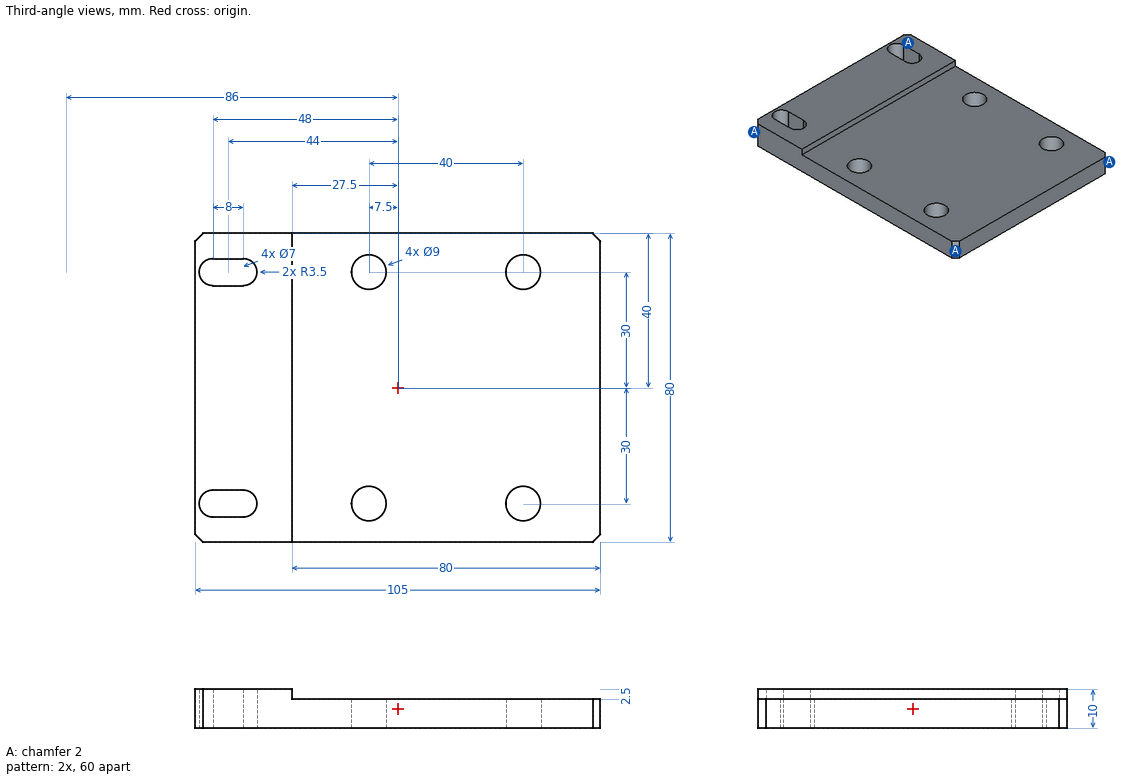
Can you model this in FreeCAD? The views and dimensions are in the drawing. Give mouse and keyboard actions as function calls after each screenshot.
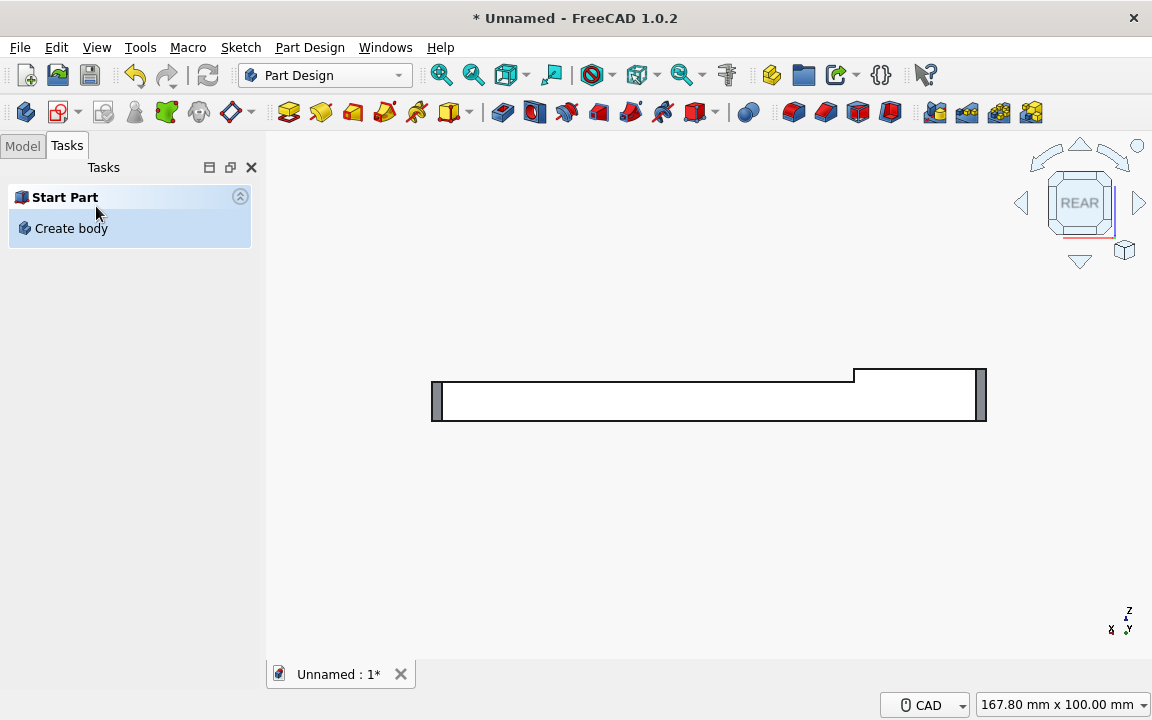
key(0)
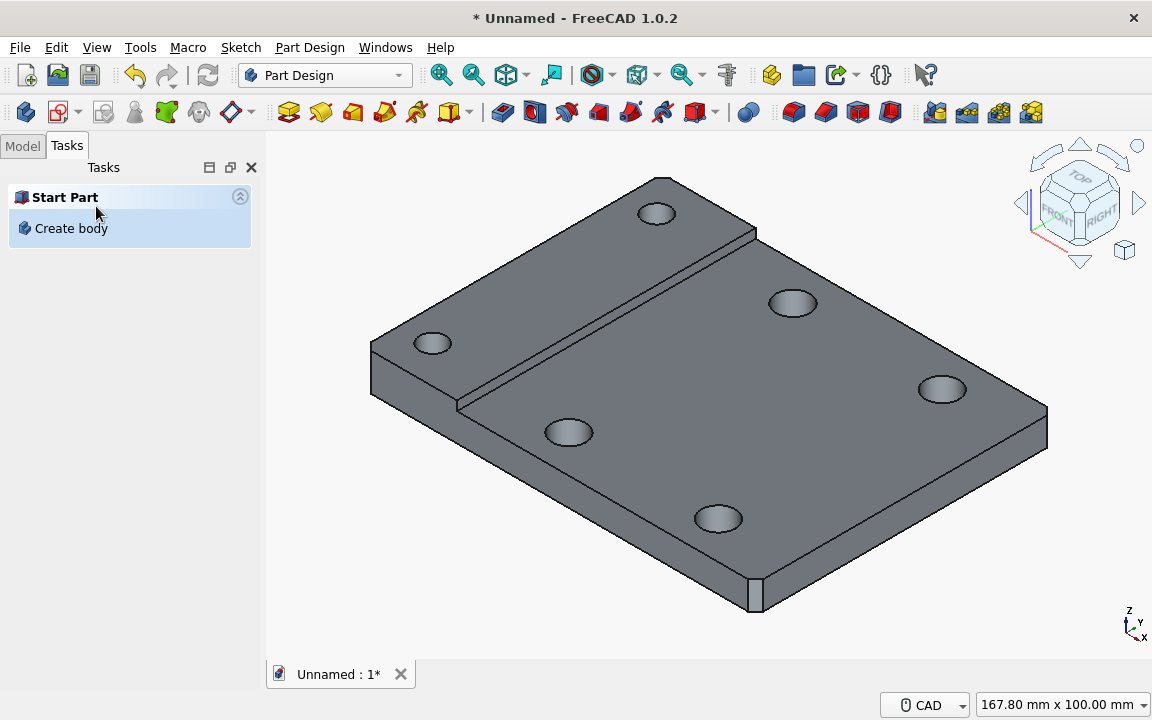
click(602, 262)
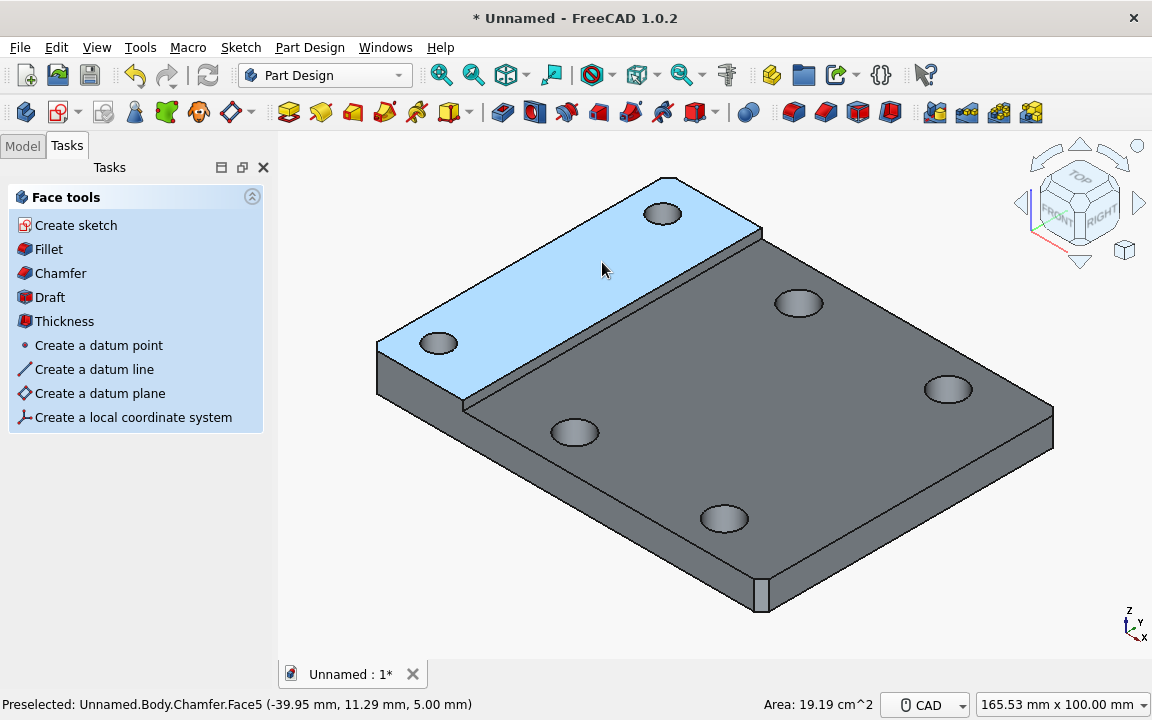
click(58, 112)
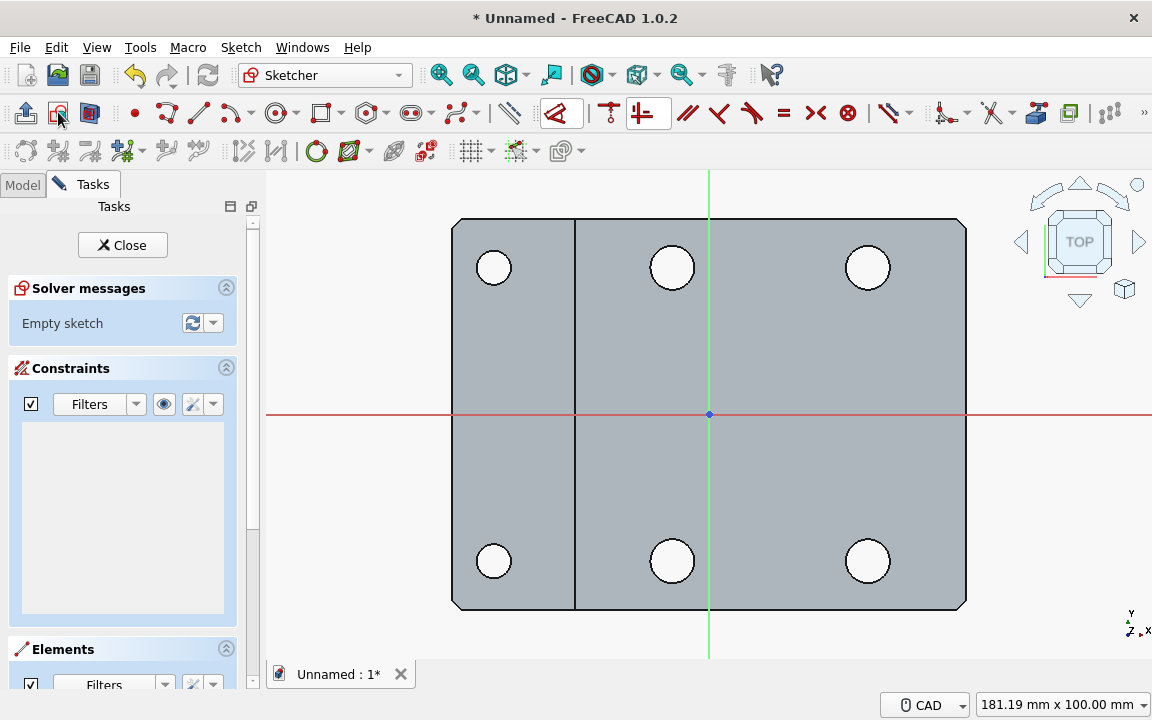
scroll(465, 239, up, 9)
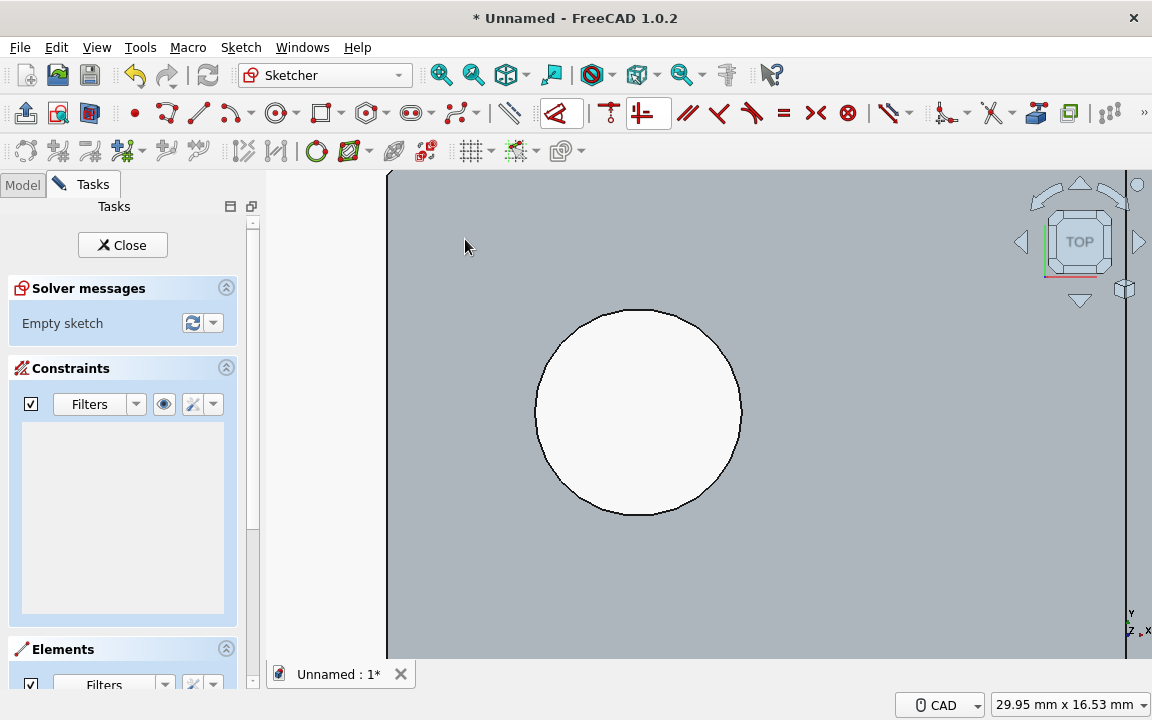
click(412, 114)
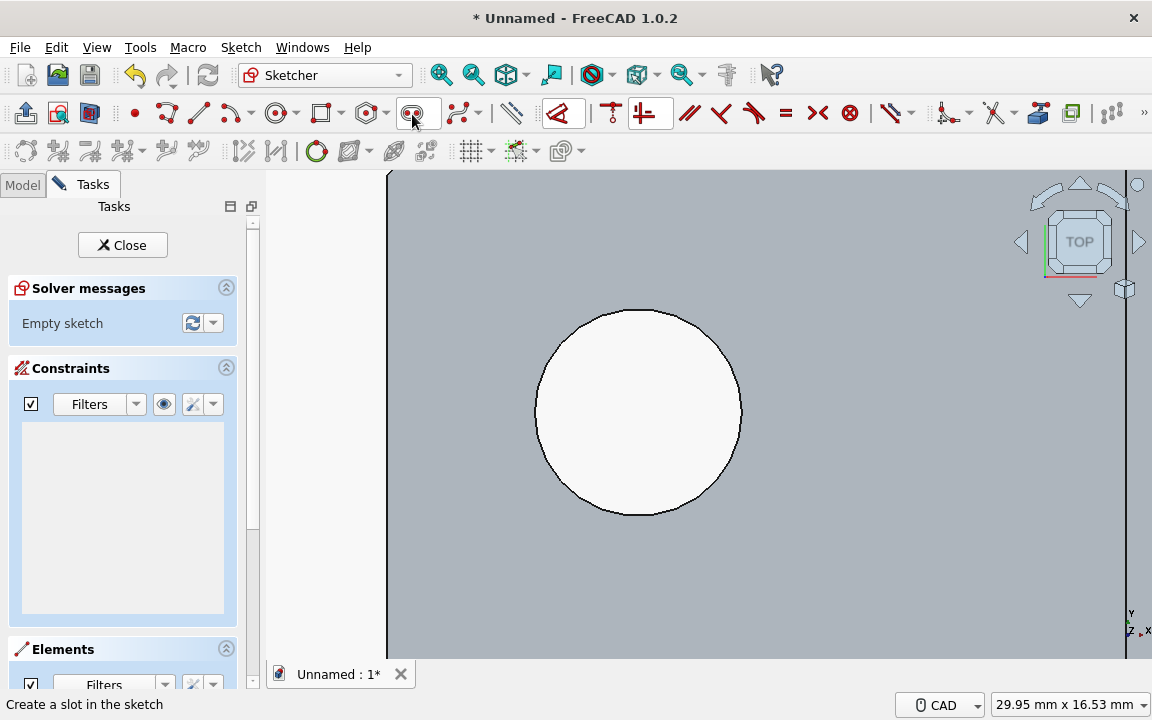
click(520, 413)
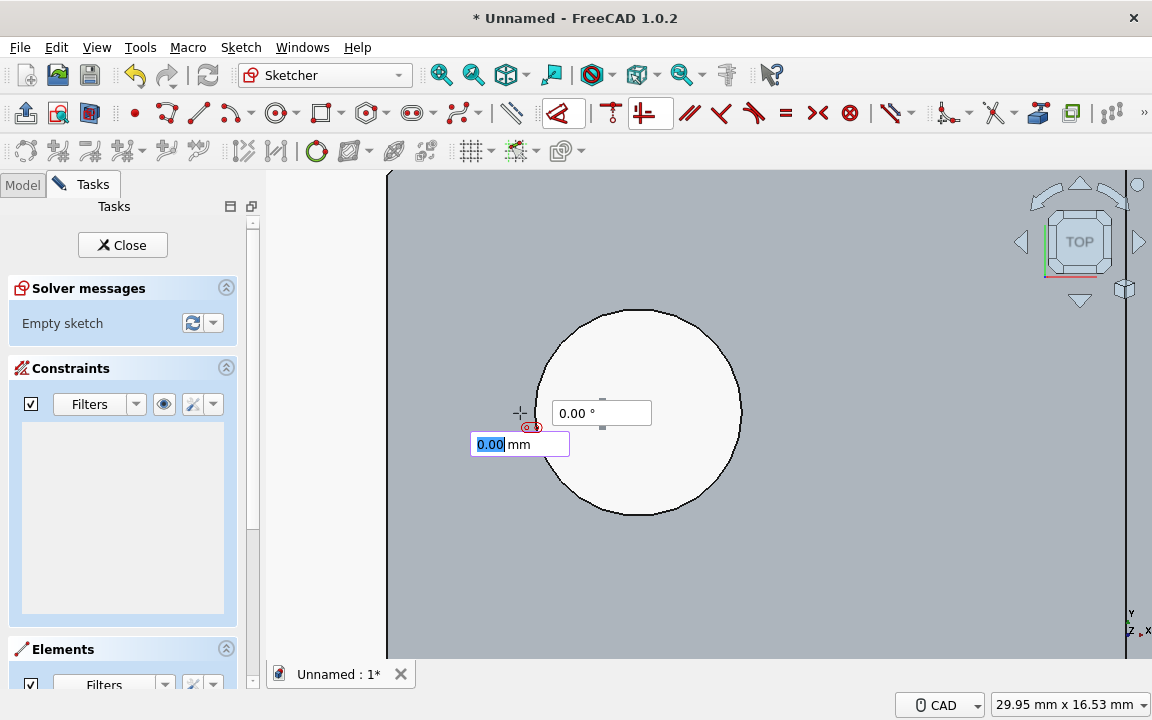
click(757, 413)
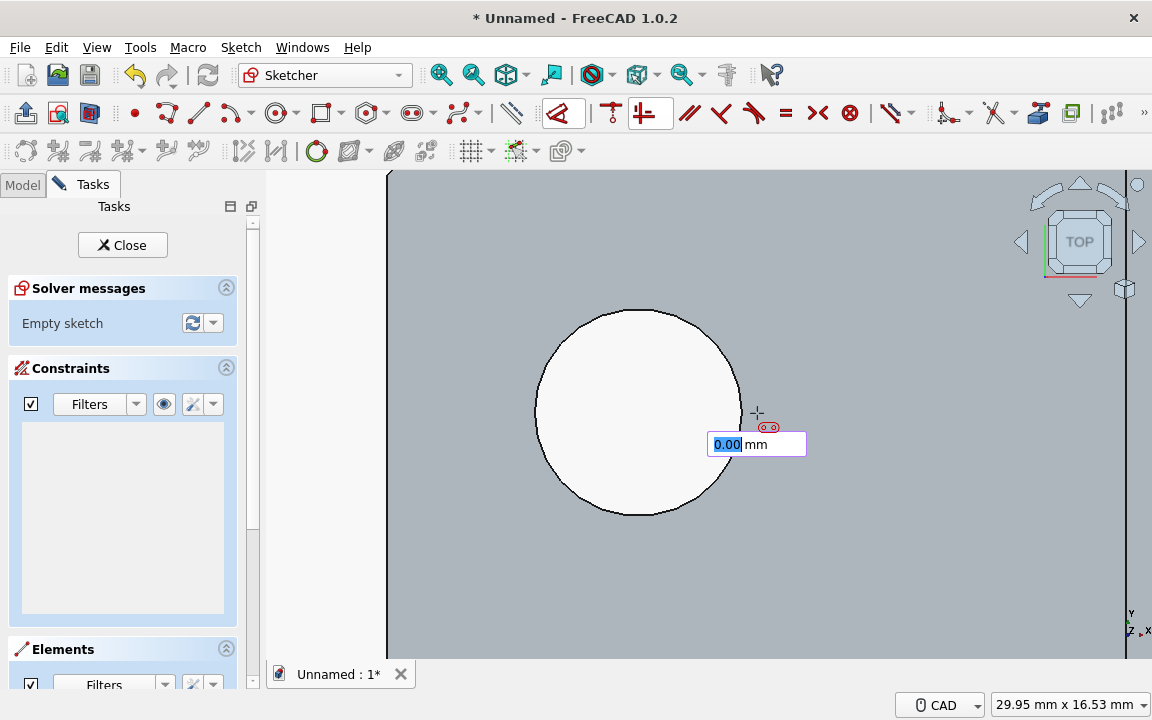
click(638, 516)
key(Escape)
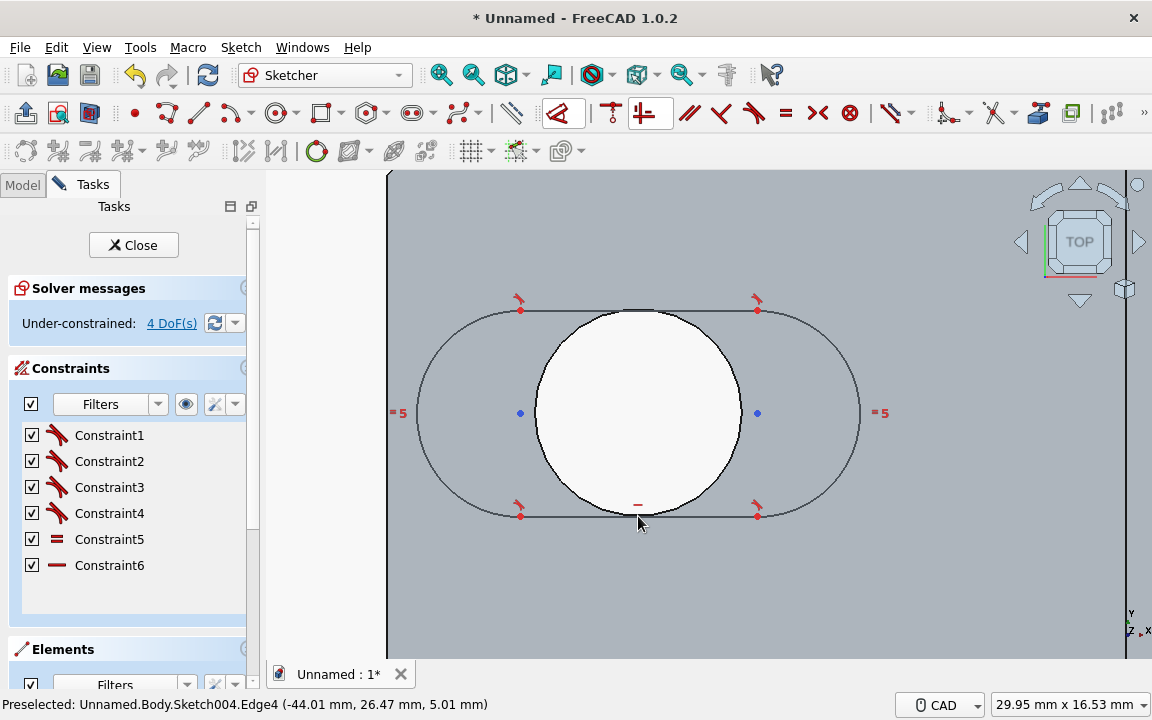
click(437, 353)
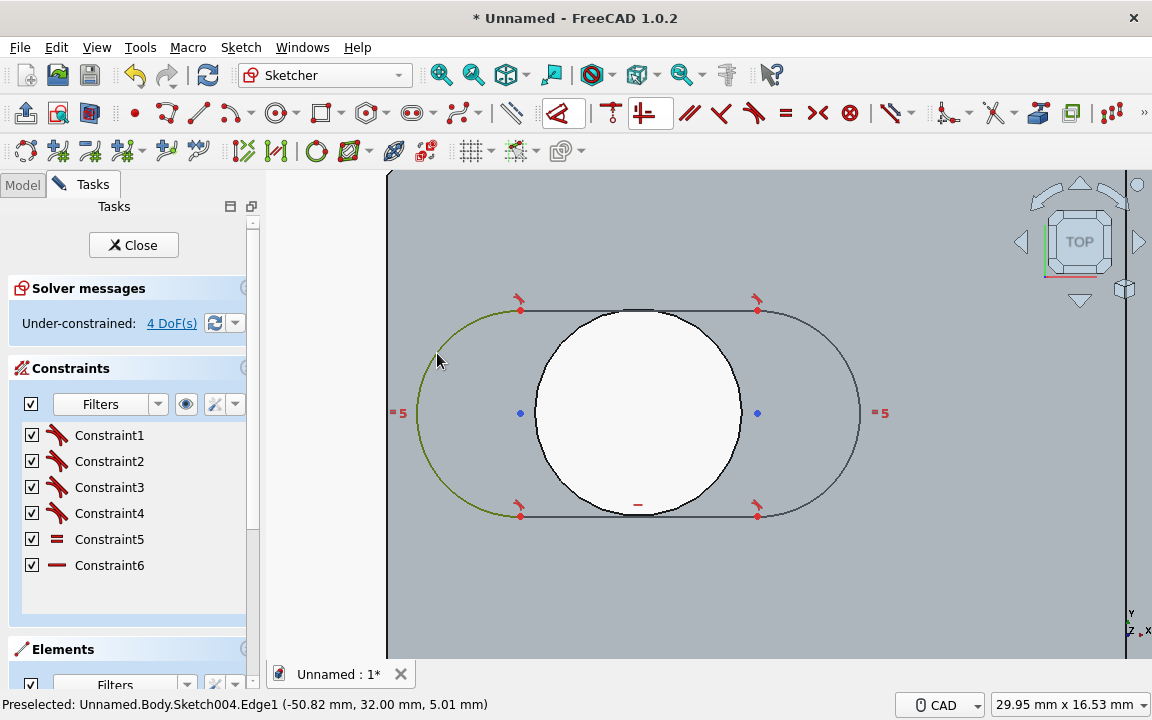
key(k)
key(r)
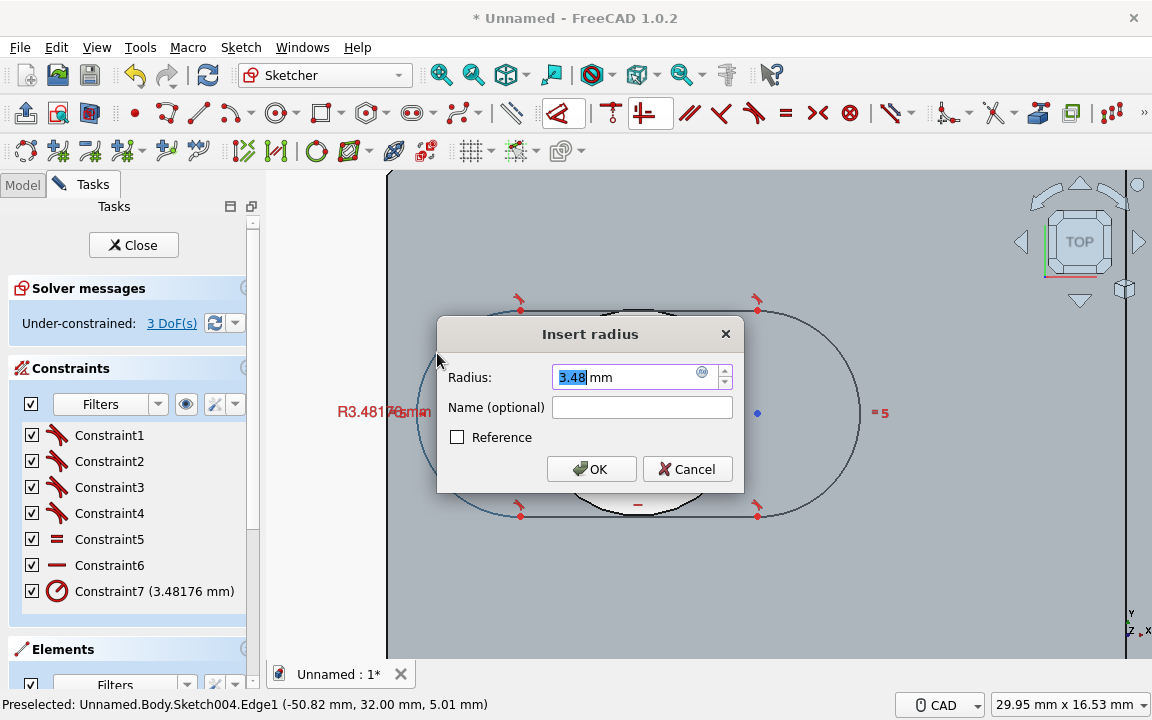
text(3.5)
key(Return)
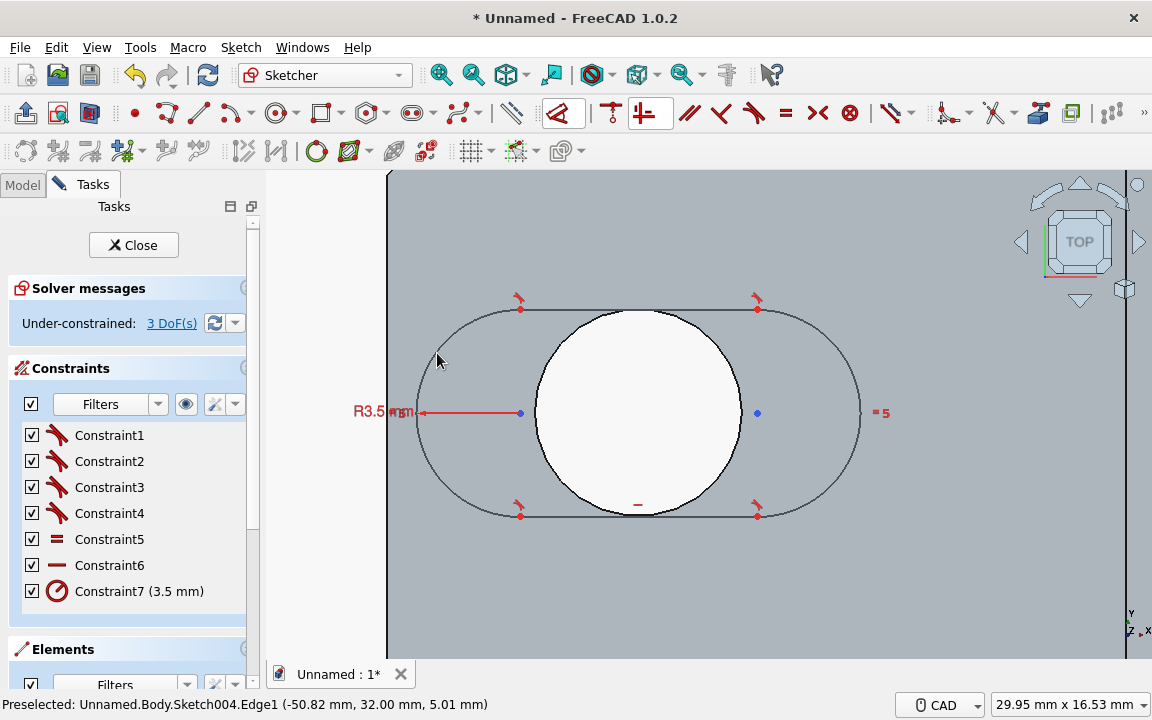
click(591, 310)